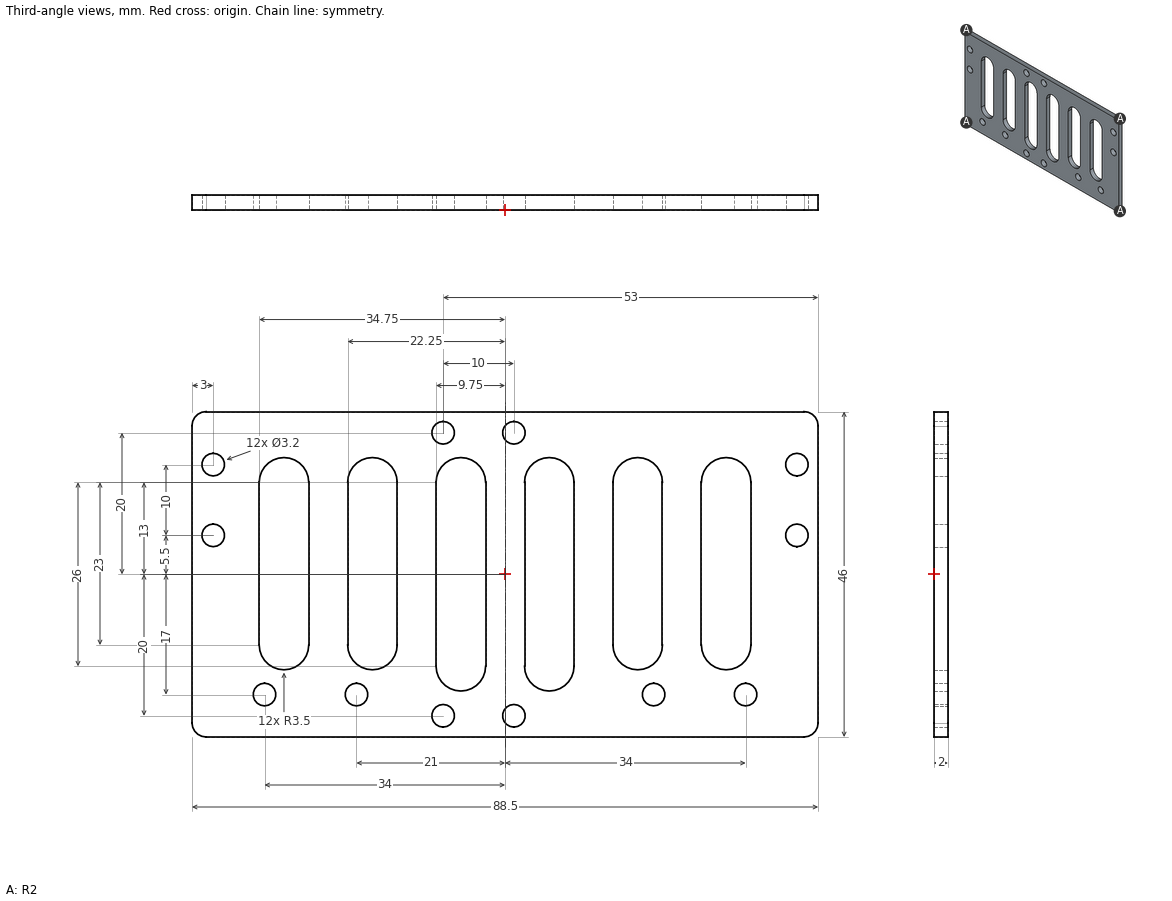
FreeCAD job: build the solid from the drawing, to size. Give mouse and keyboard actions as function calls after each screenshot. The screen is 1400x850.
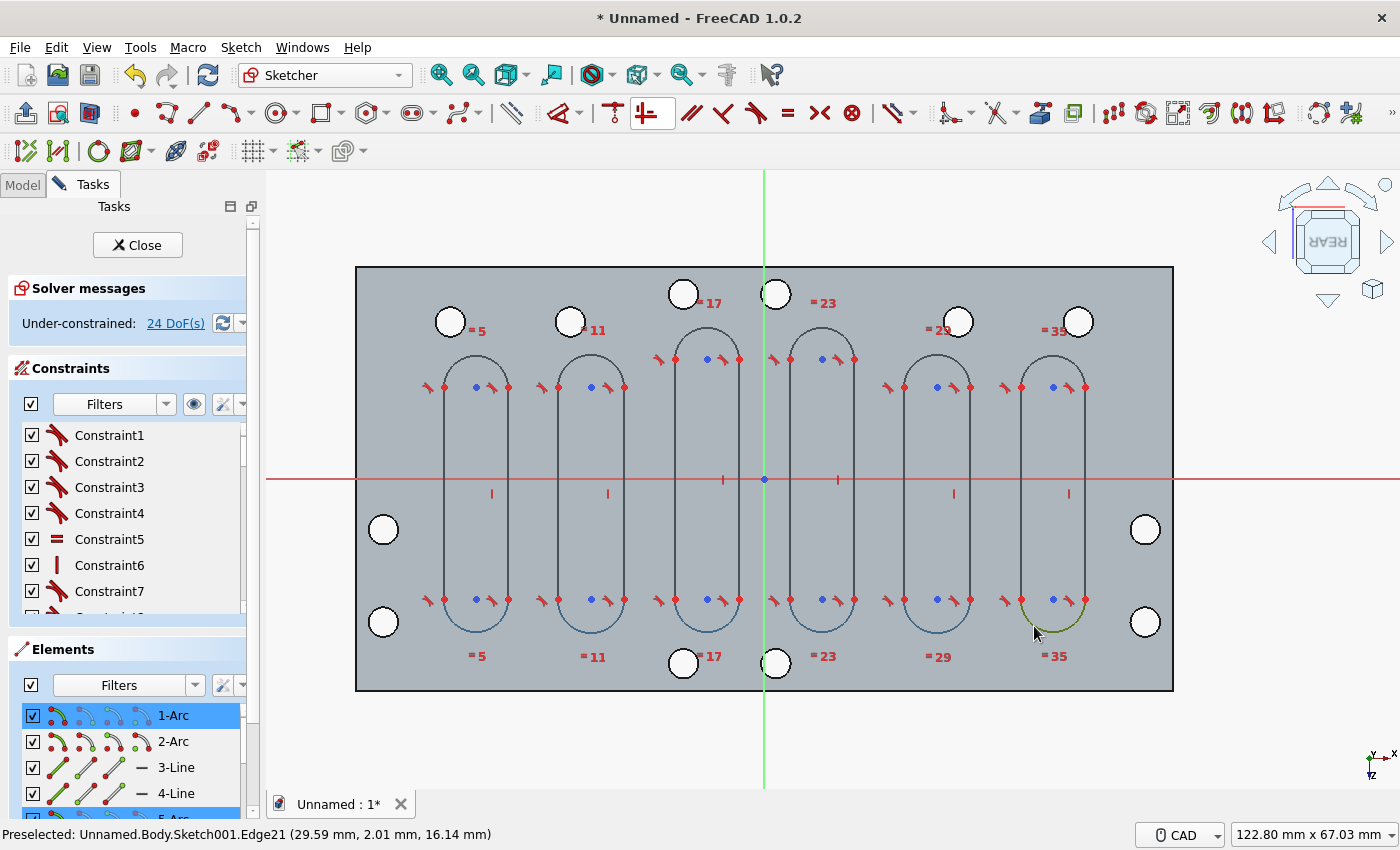
click(788, 114)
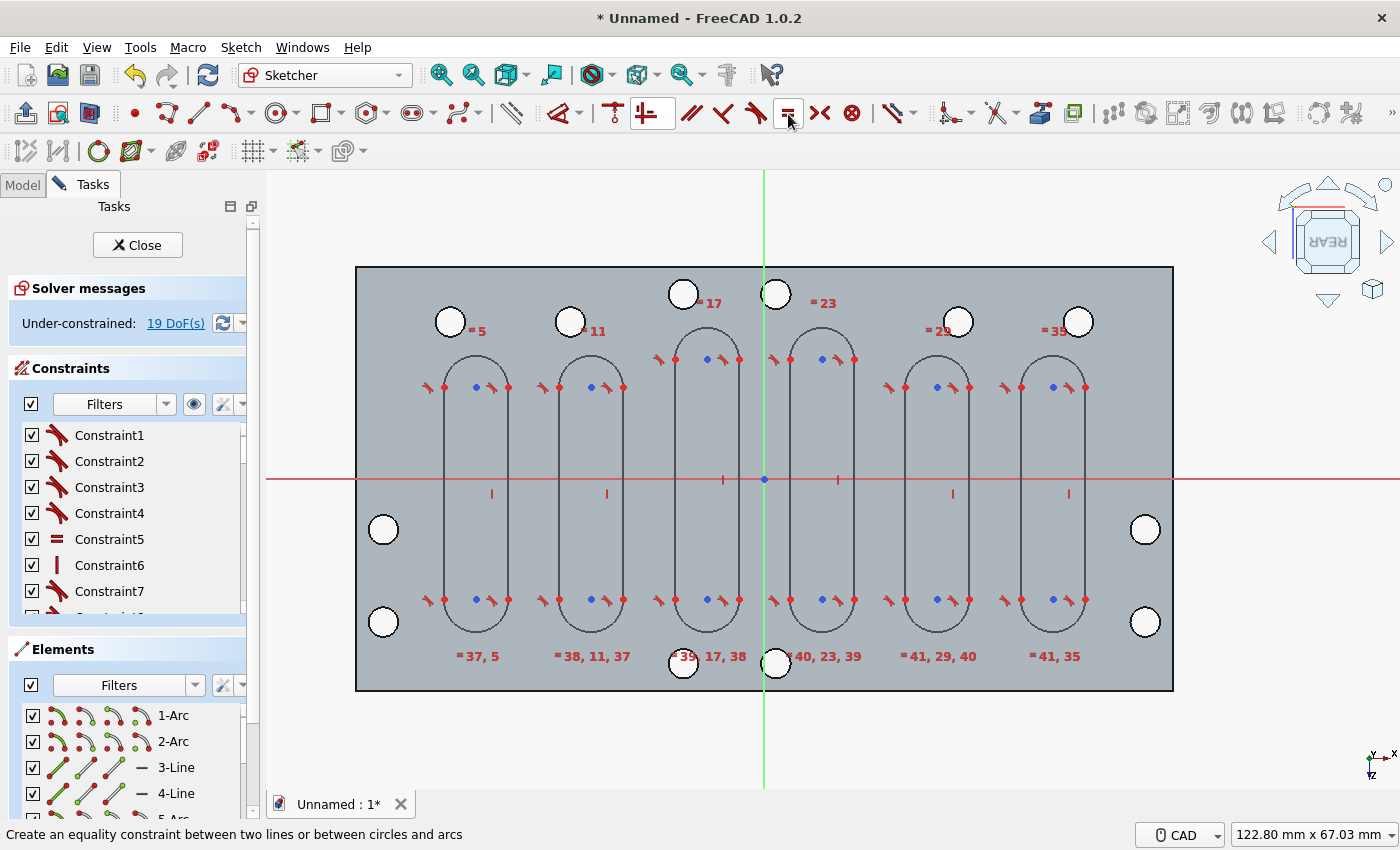
click(707, 600)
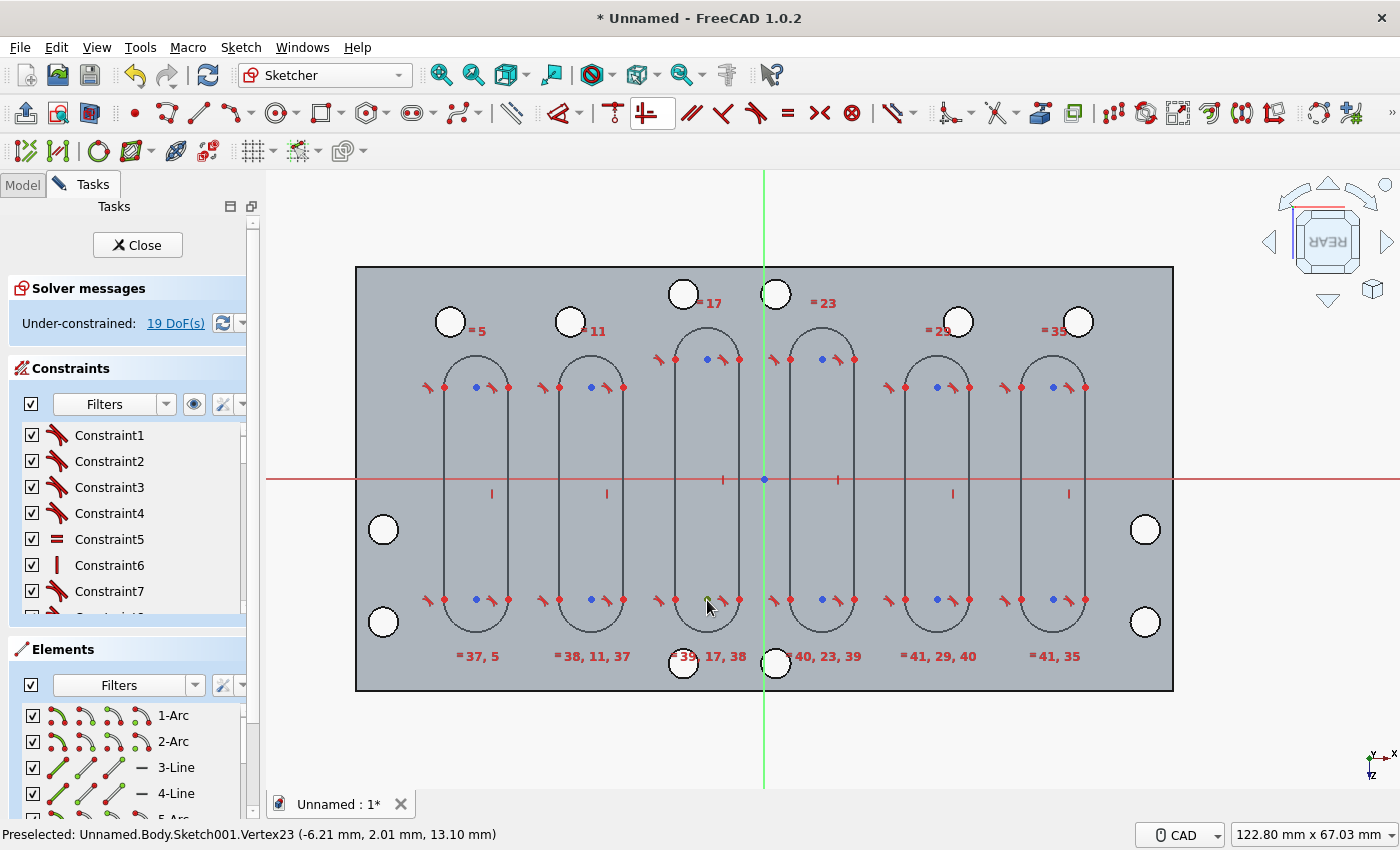
click(822, 600)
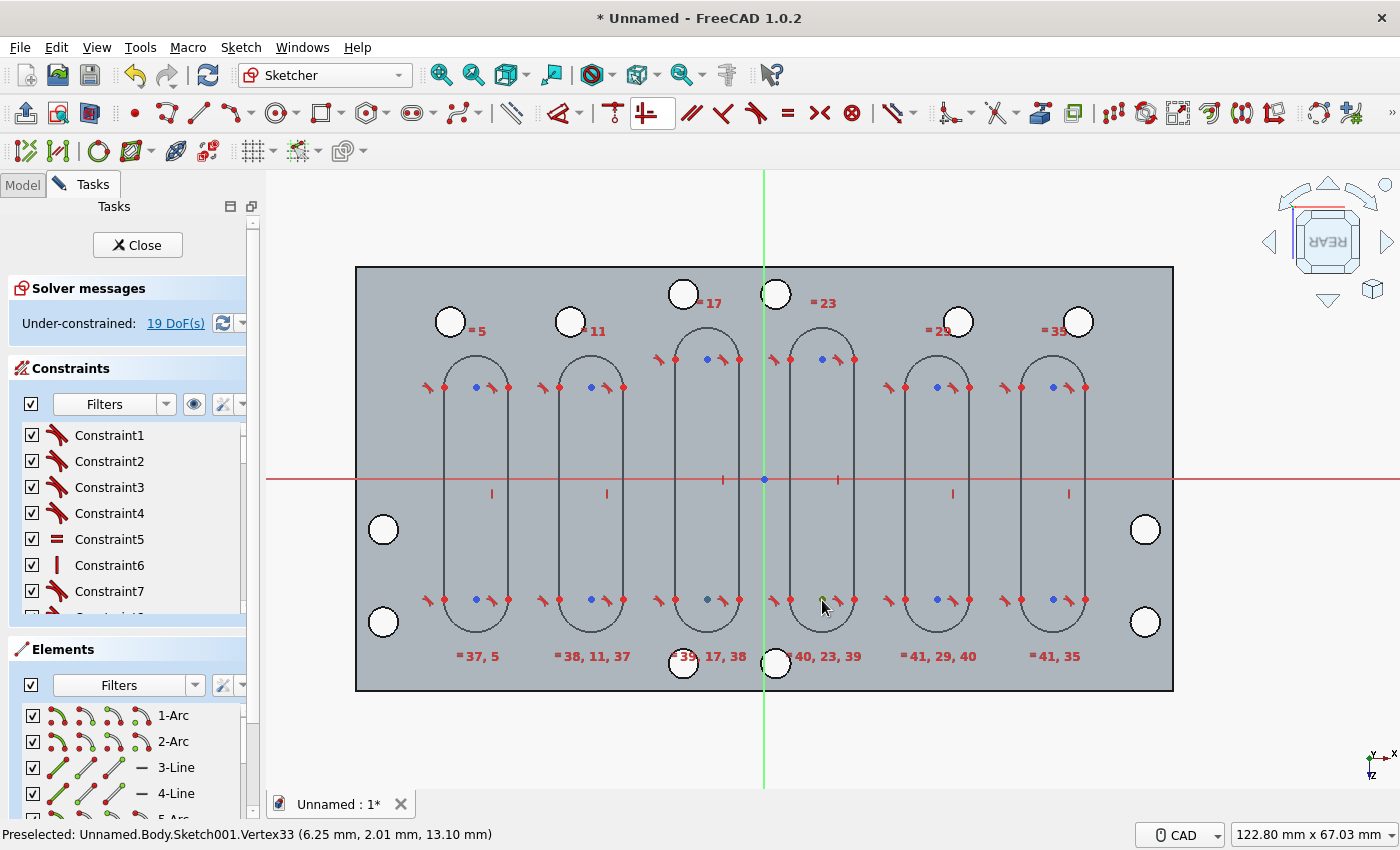
click(764, 721)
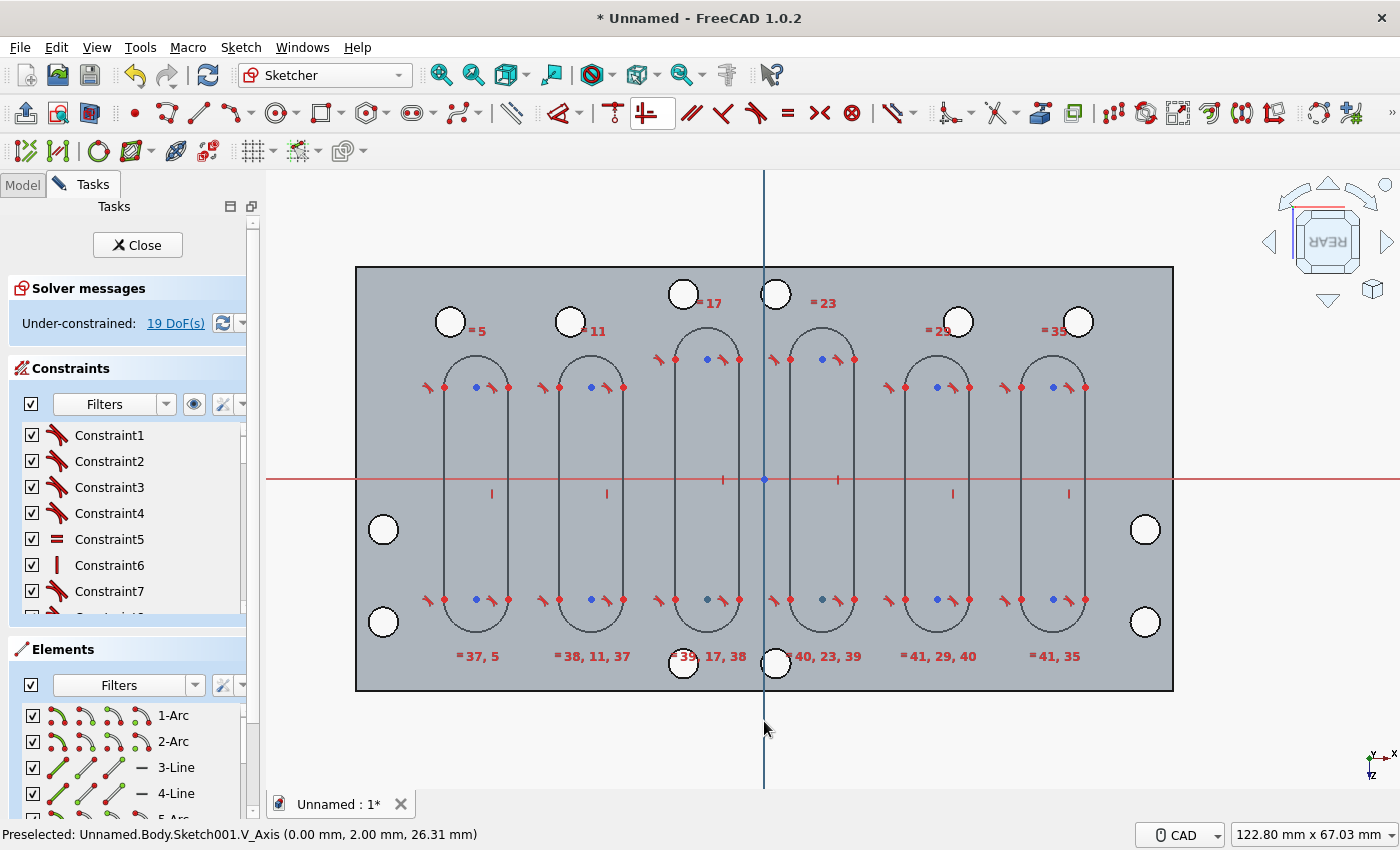
click(820, 114)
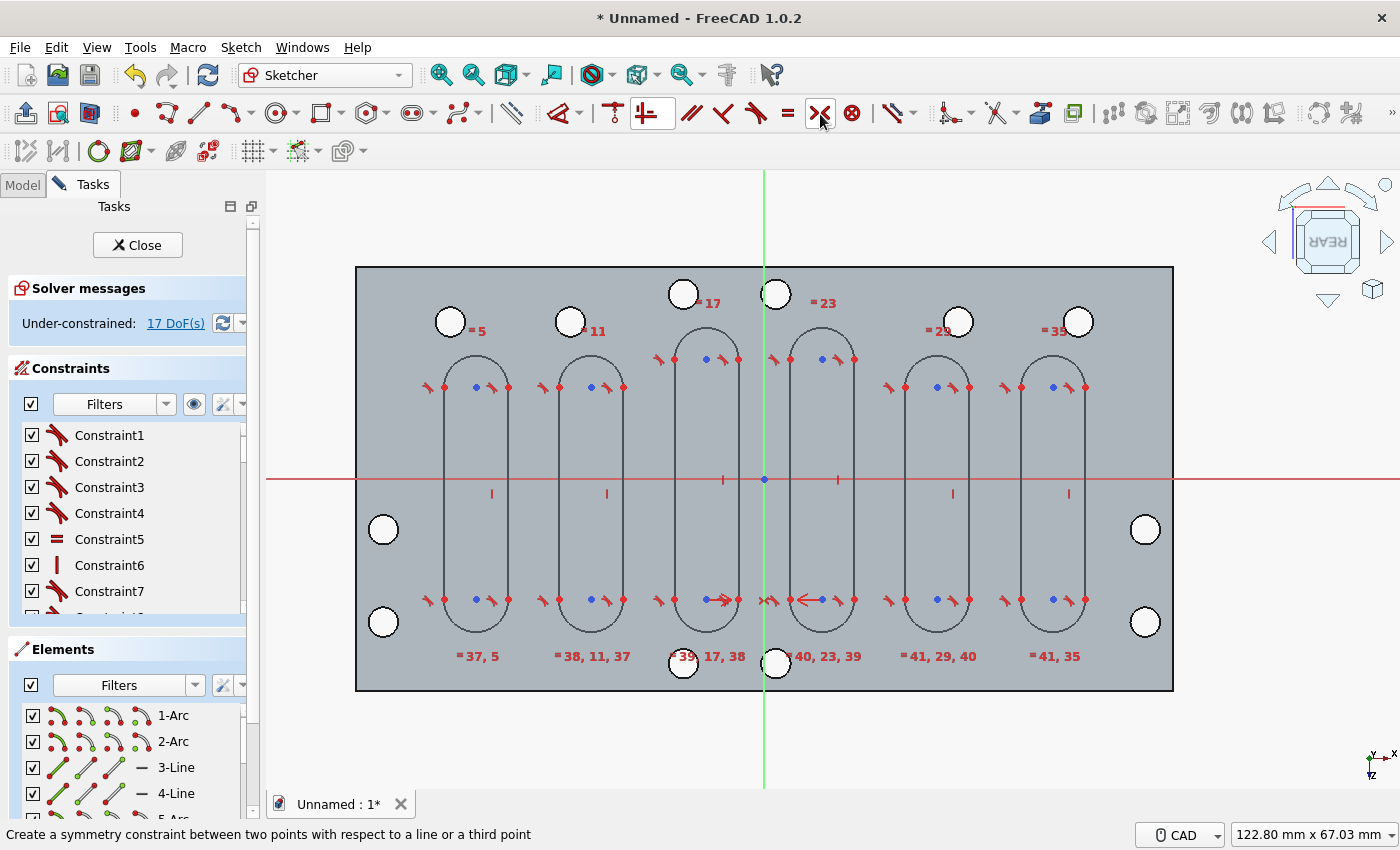
click(591, 600)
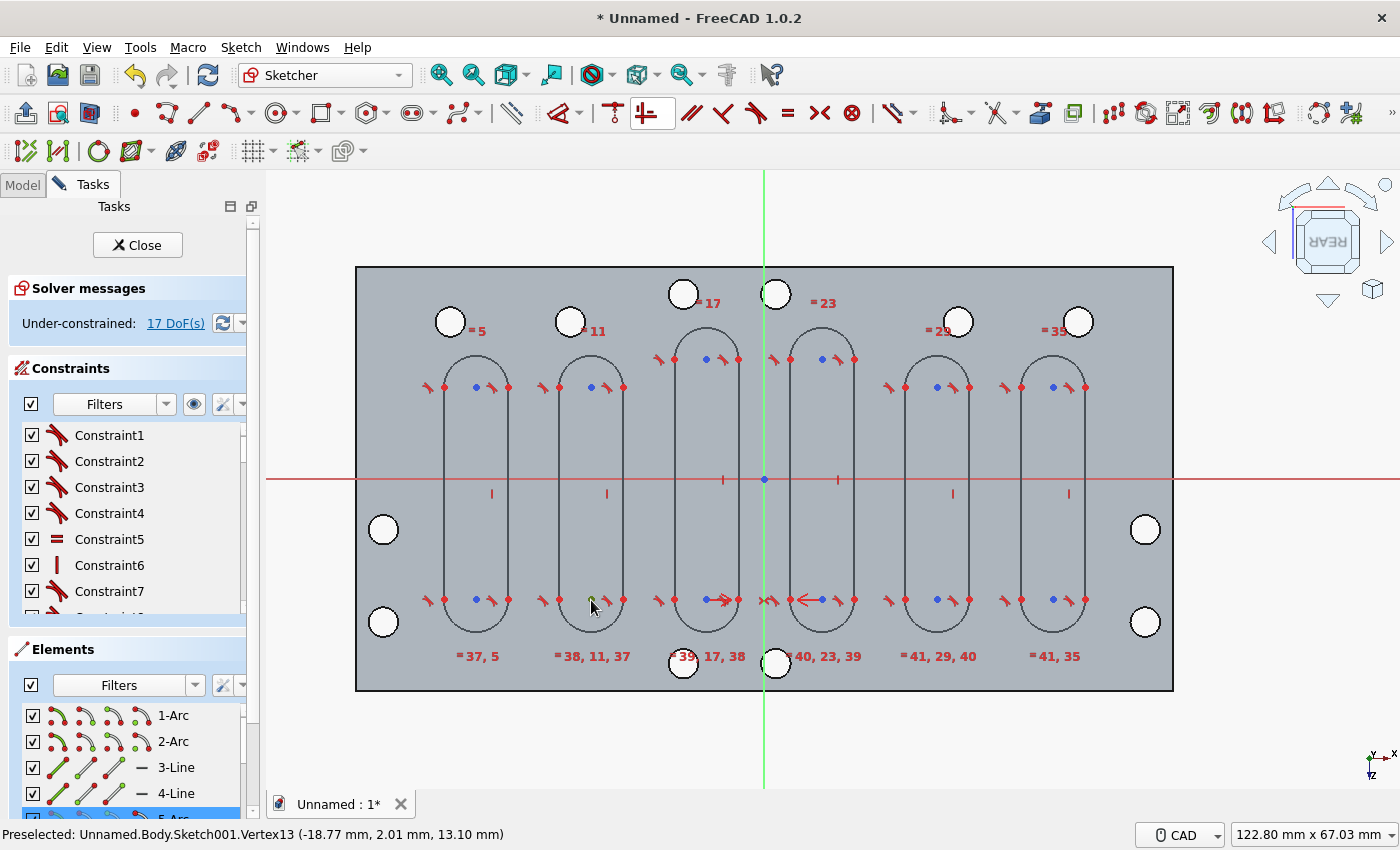
click(937, 600)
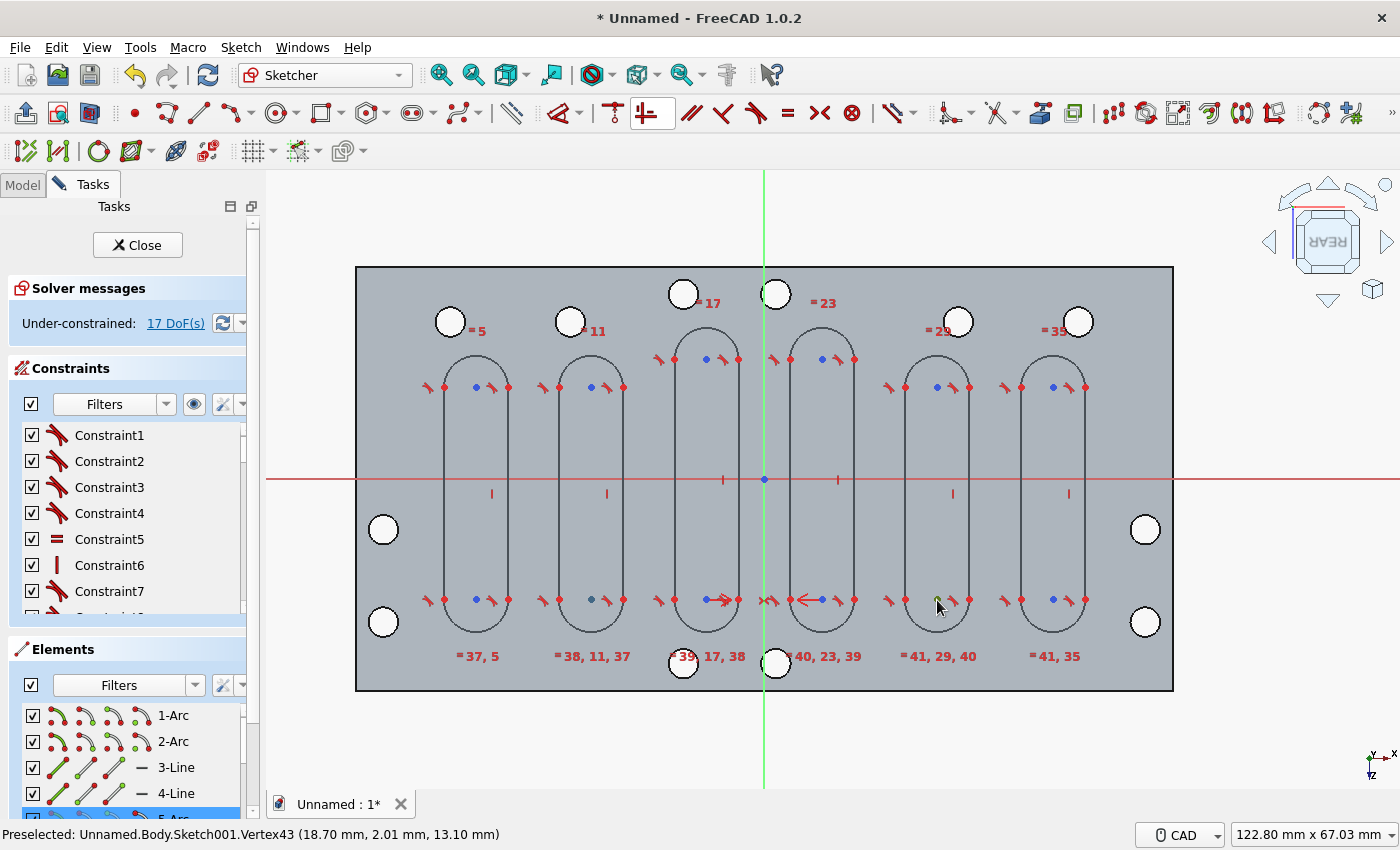
click(764, 721)